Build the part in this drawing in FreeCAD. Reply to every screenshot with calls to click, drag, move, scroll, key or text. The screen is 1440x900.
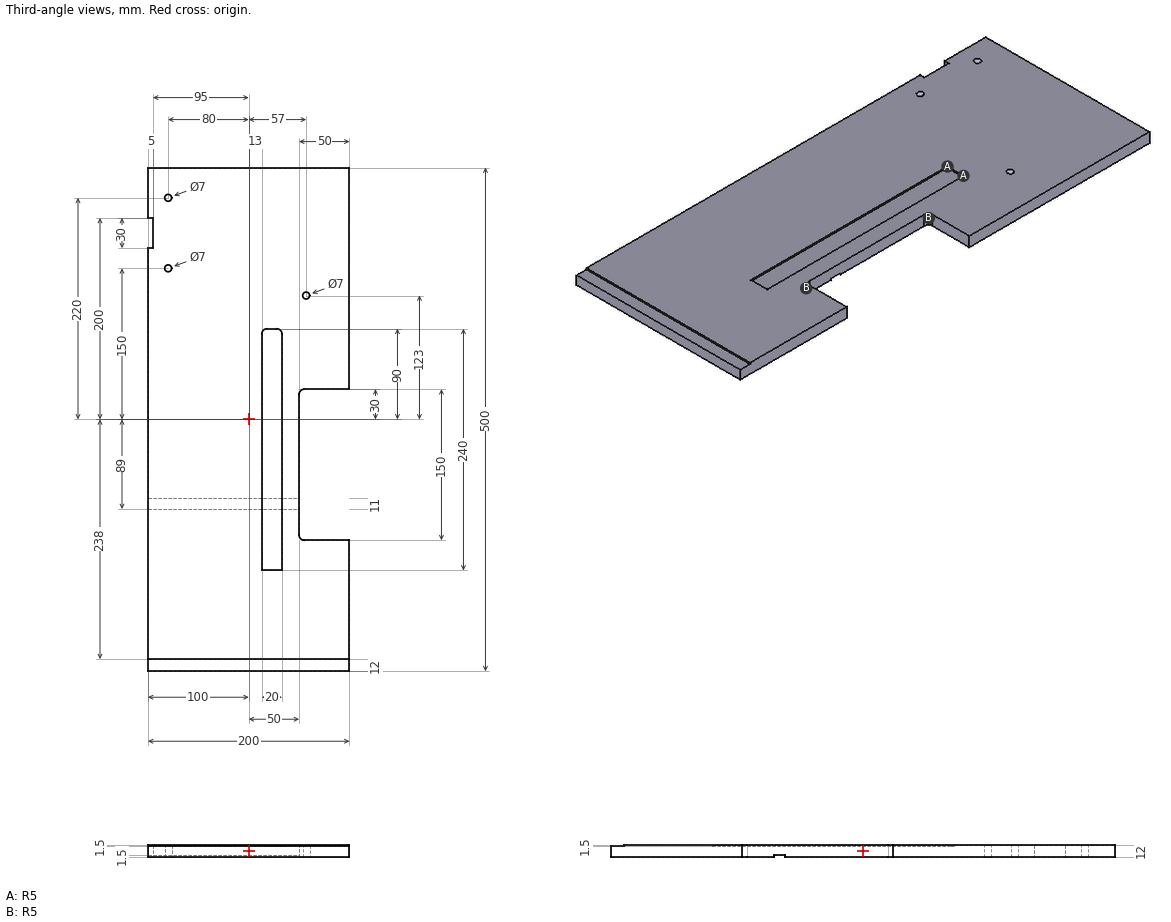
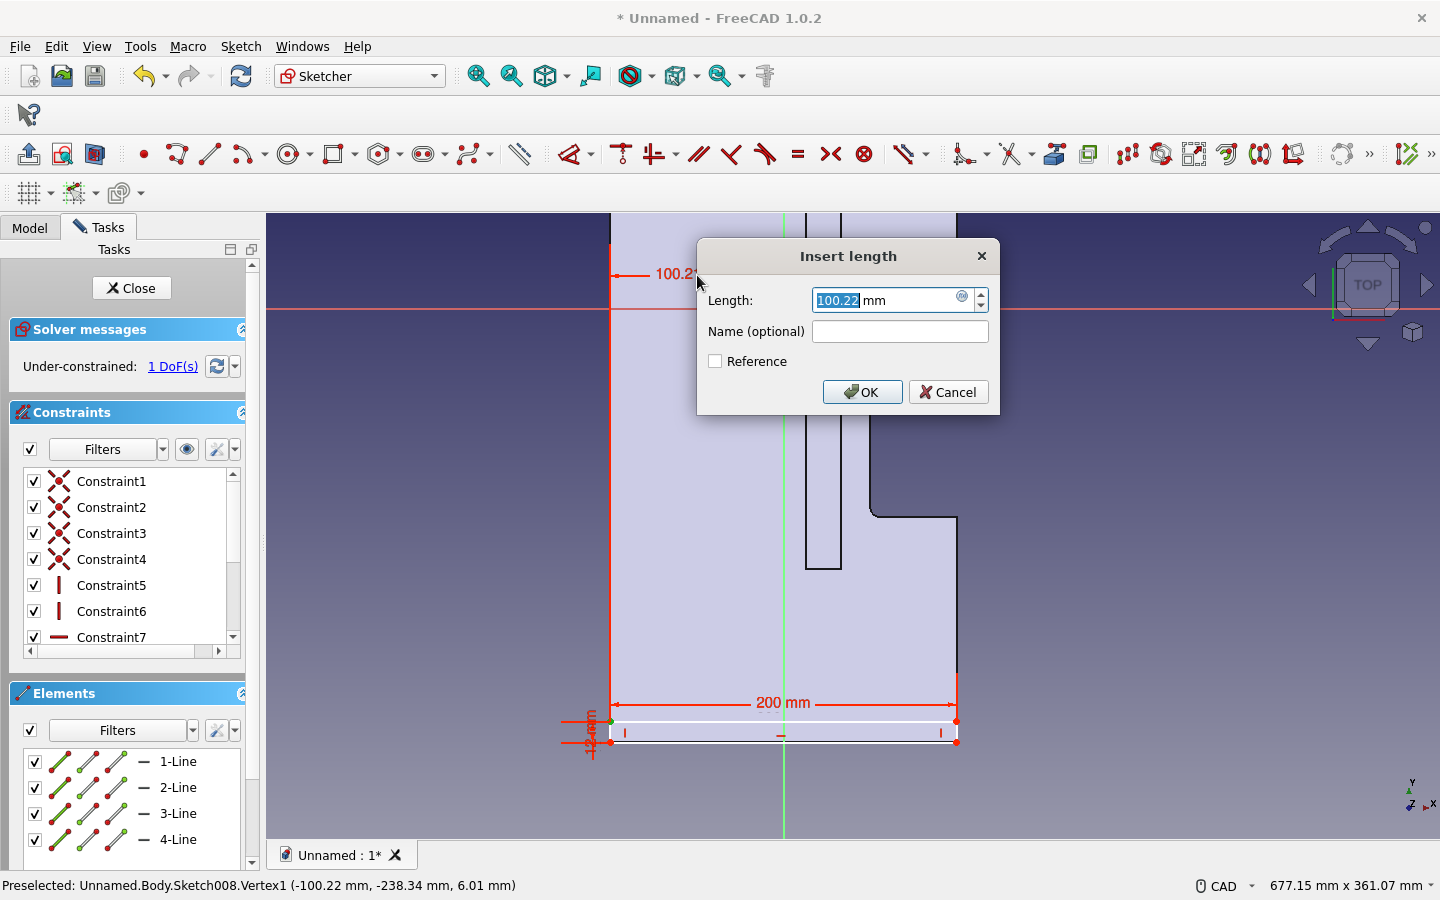
text(100)
key(Return)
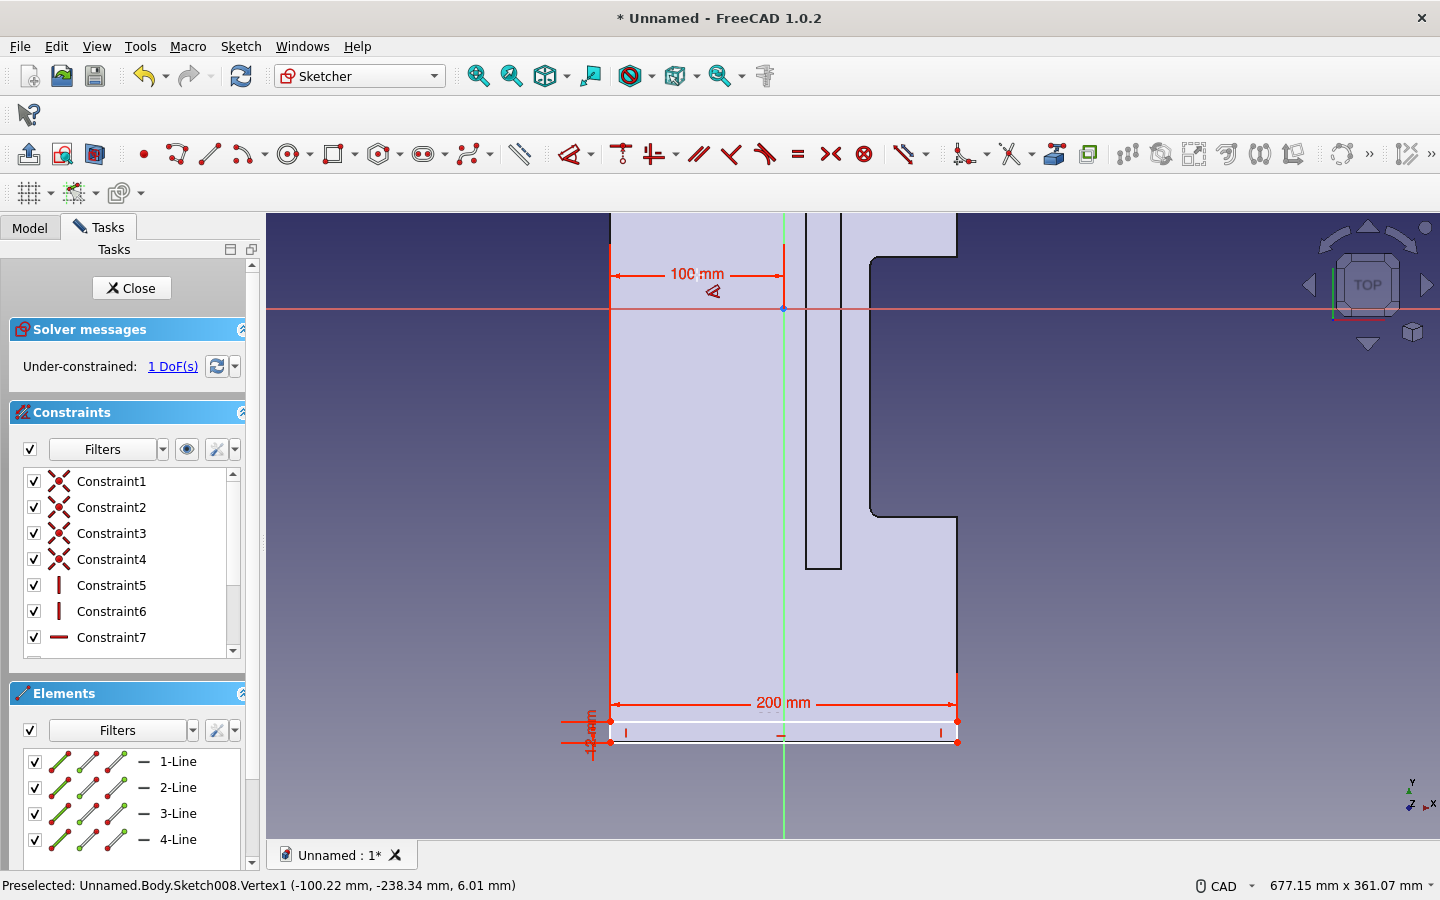
click(610, 722)
click(576, 515)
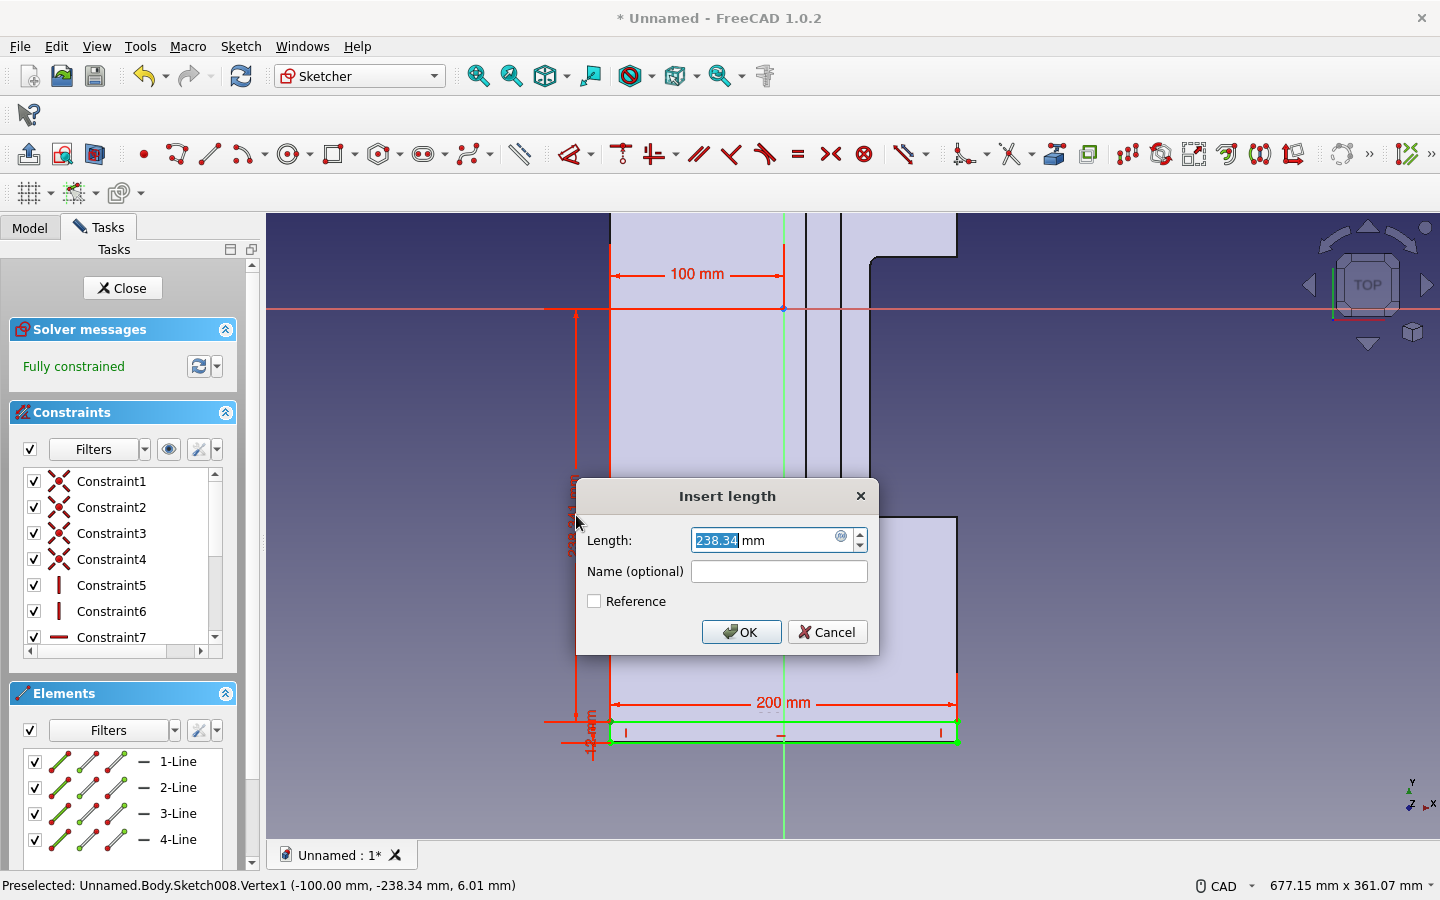
text(238)
key(Return)
key(Escape)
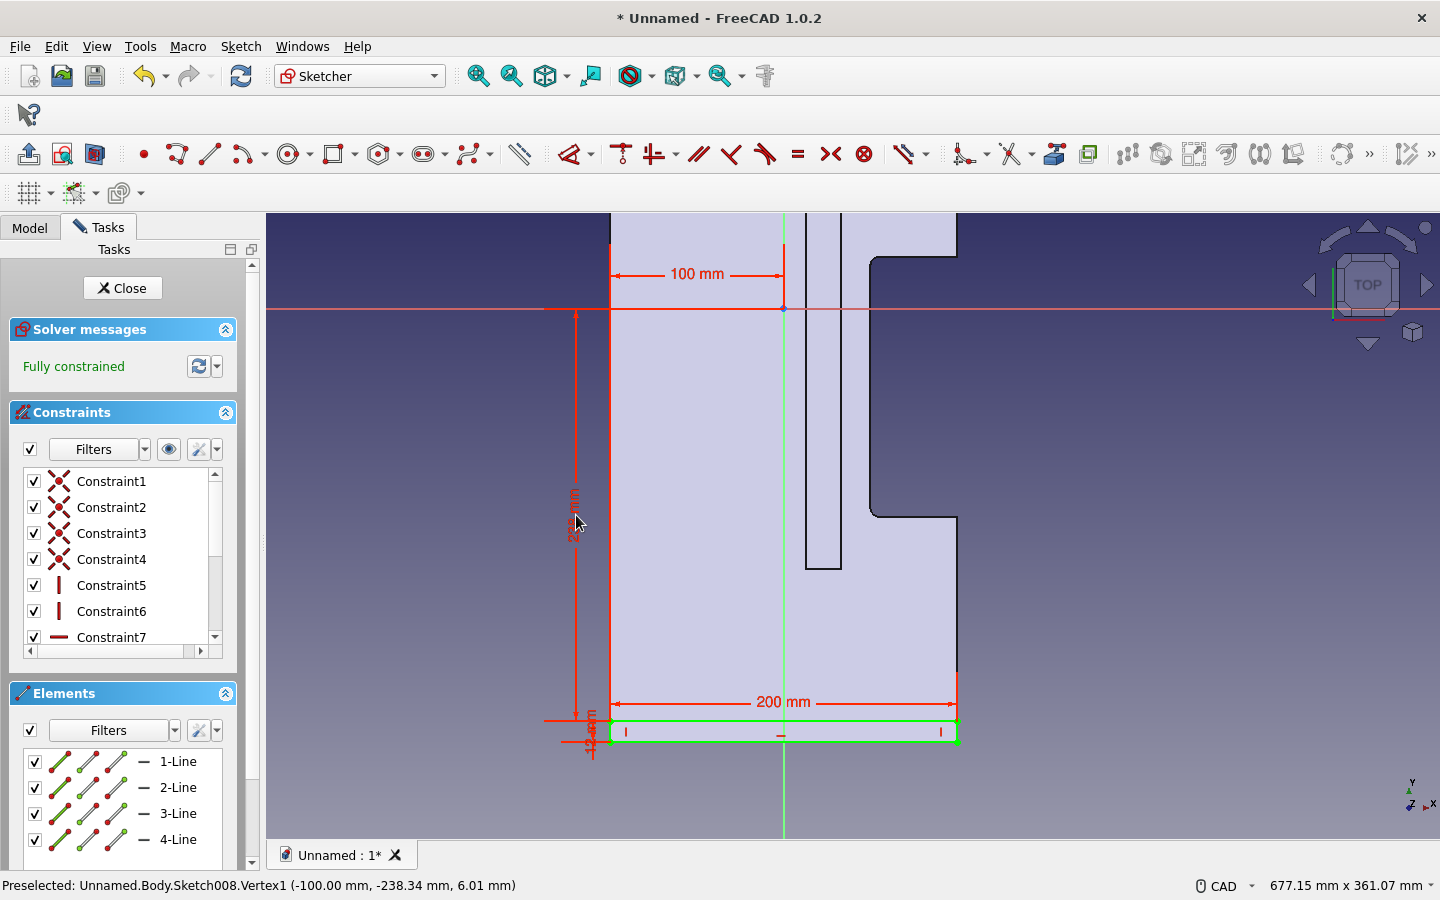
click(123, 288)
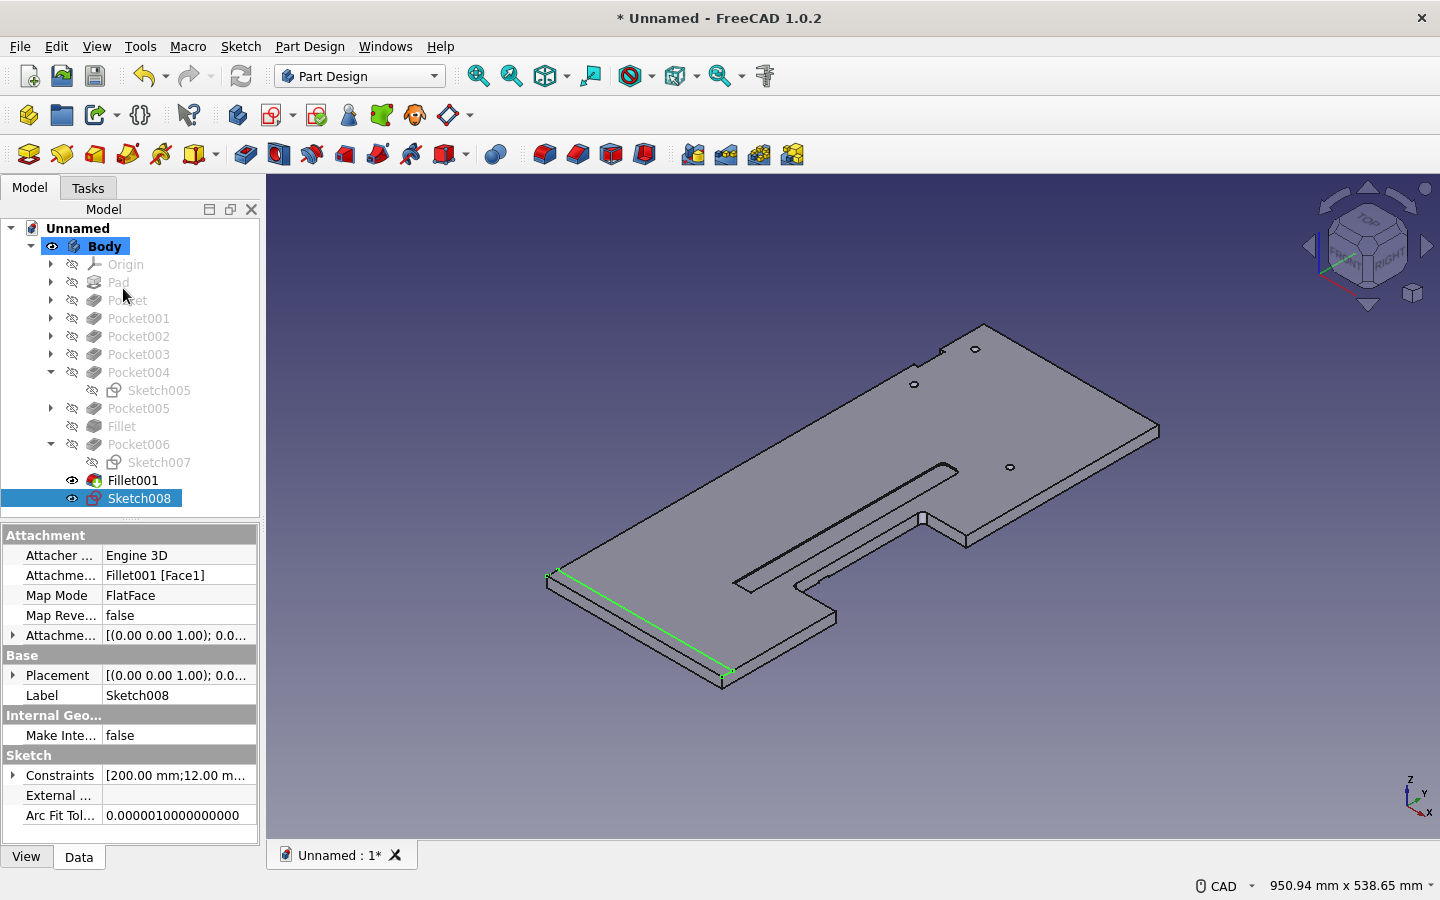
click(246, 154)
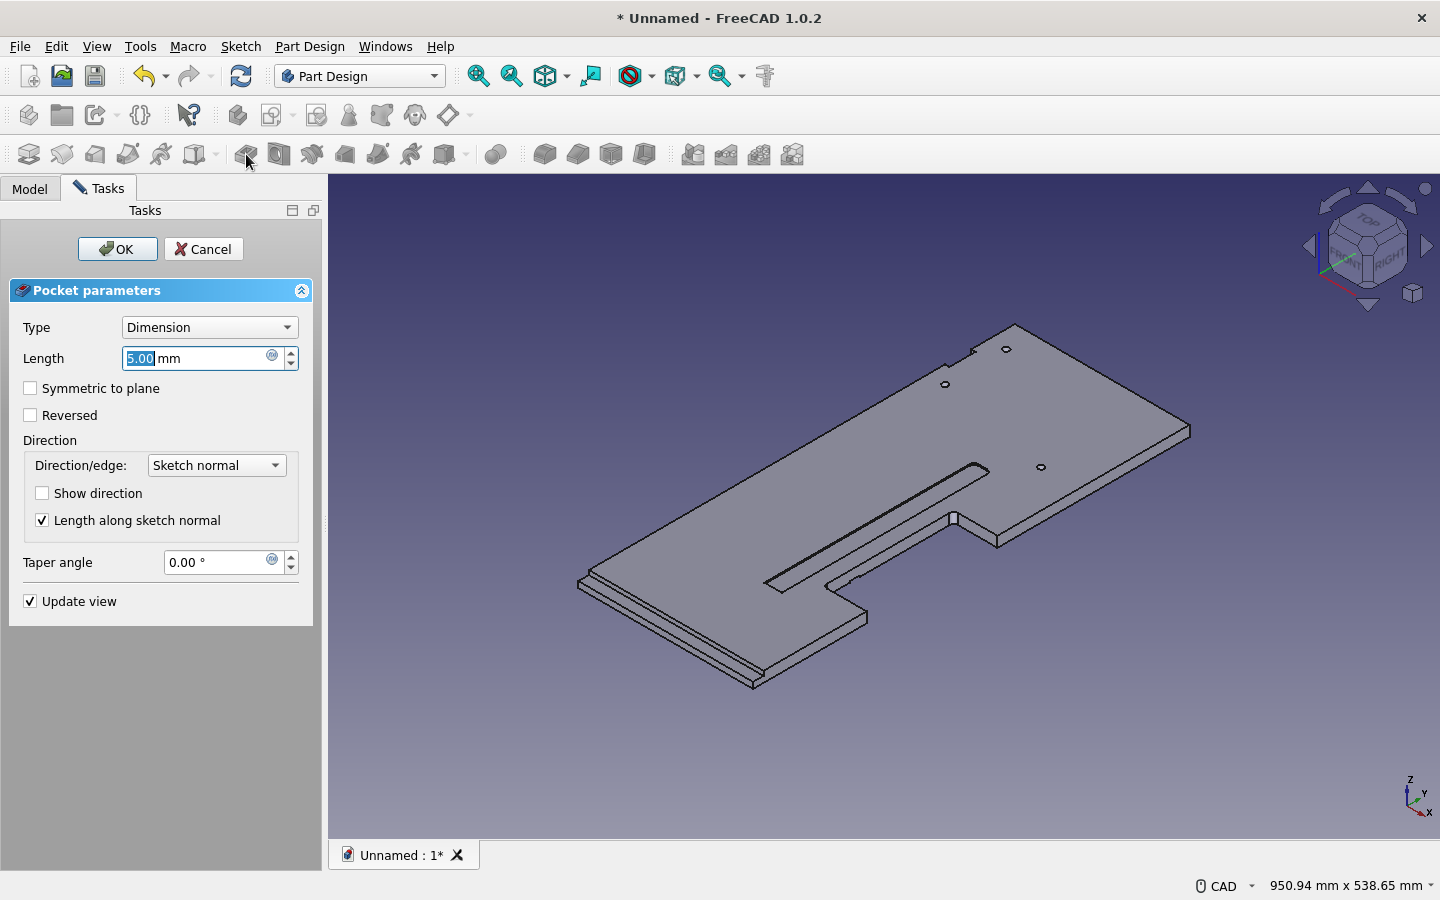
text(1.5)
key(Tab)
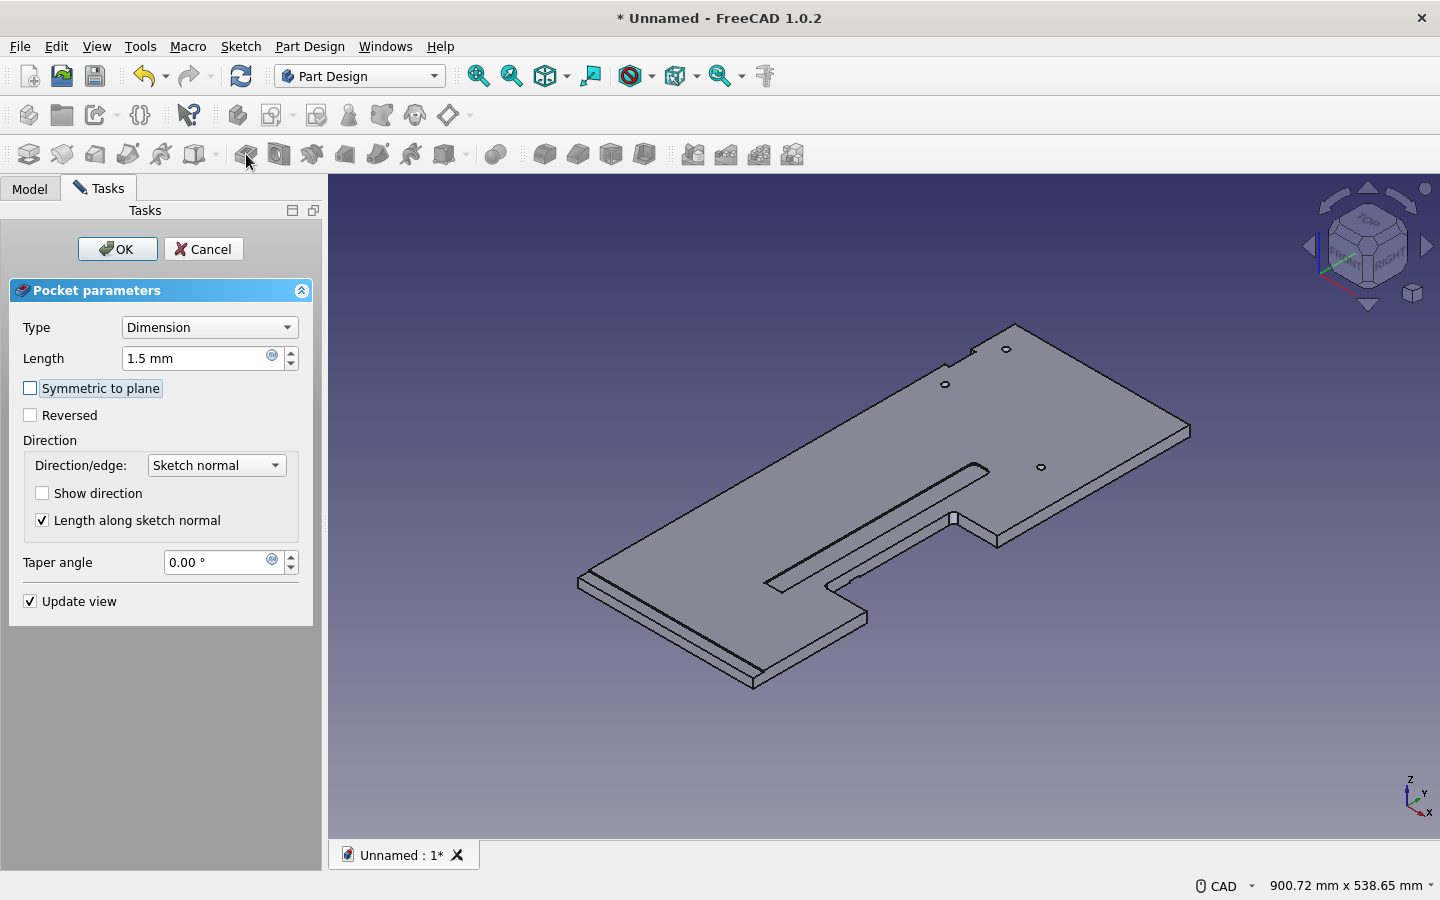
click(118, 249)